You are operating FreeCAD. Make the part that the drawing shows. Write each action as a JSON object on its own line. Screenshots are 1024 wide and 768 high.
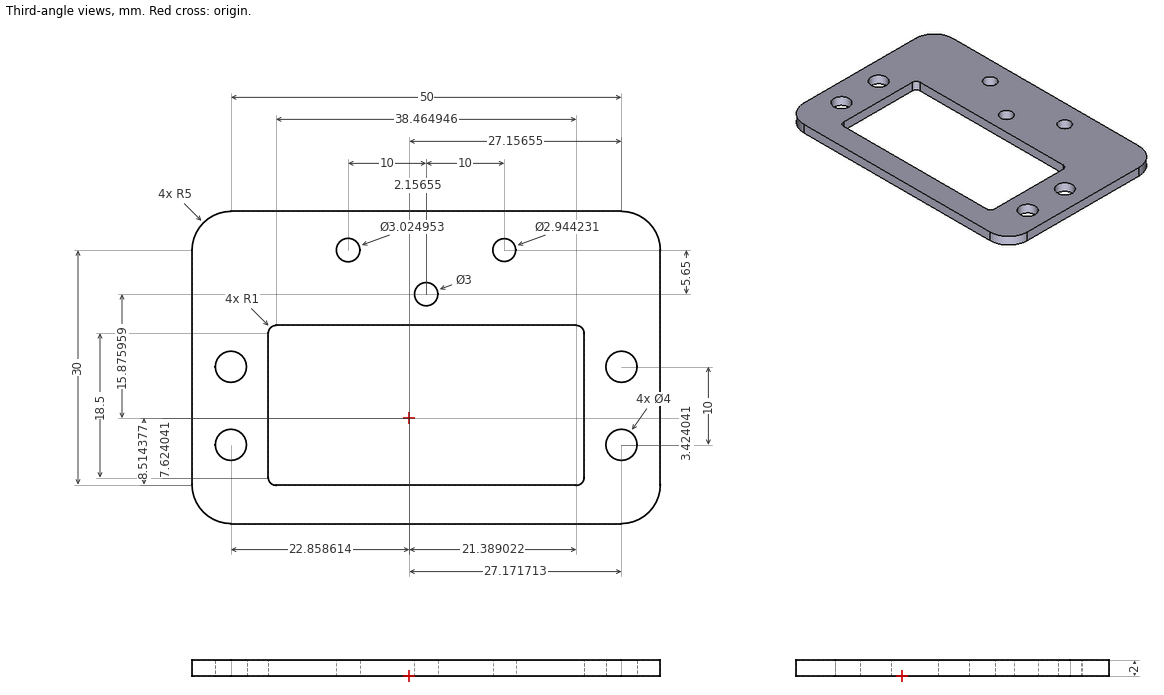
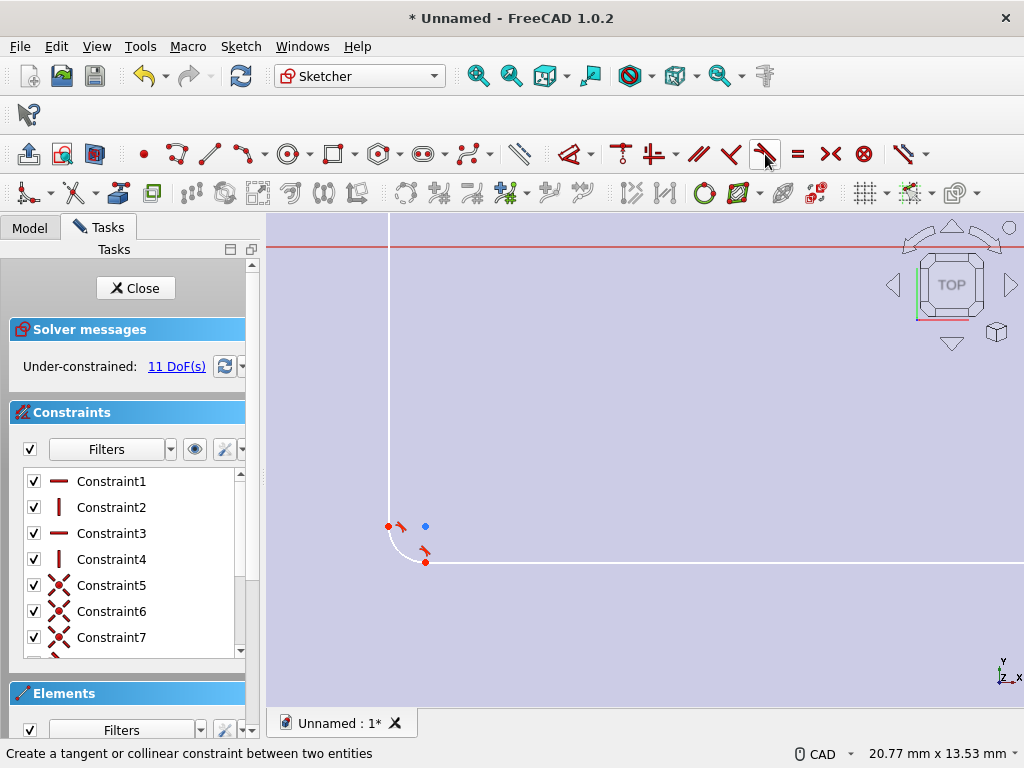
{"action": "scroll", "coordinate": [397, 549], "scroll_direction": "down", "scroll_amount": 7}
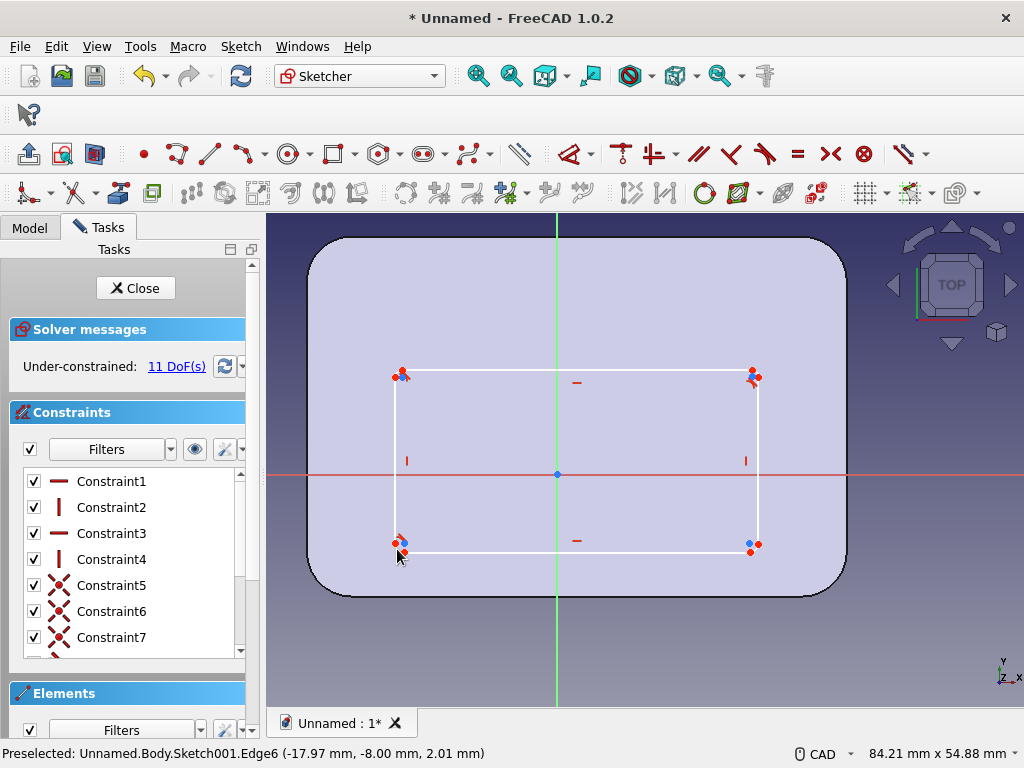
{"action": "left_click", "coordinate": [508, 553]}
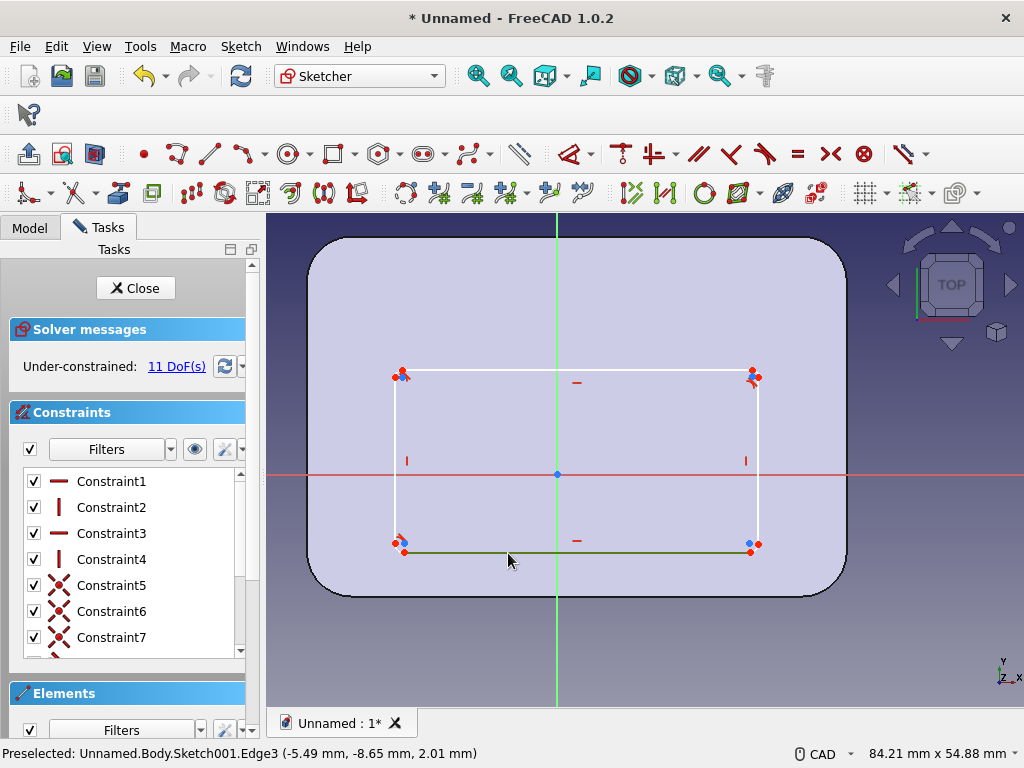
{"action": "scroll", "coordinate": [756, 550], "scroll_direction": "up", "scroll_amount": 4}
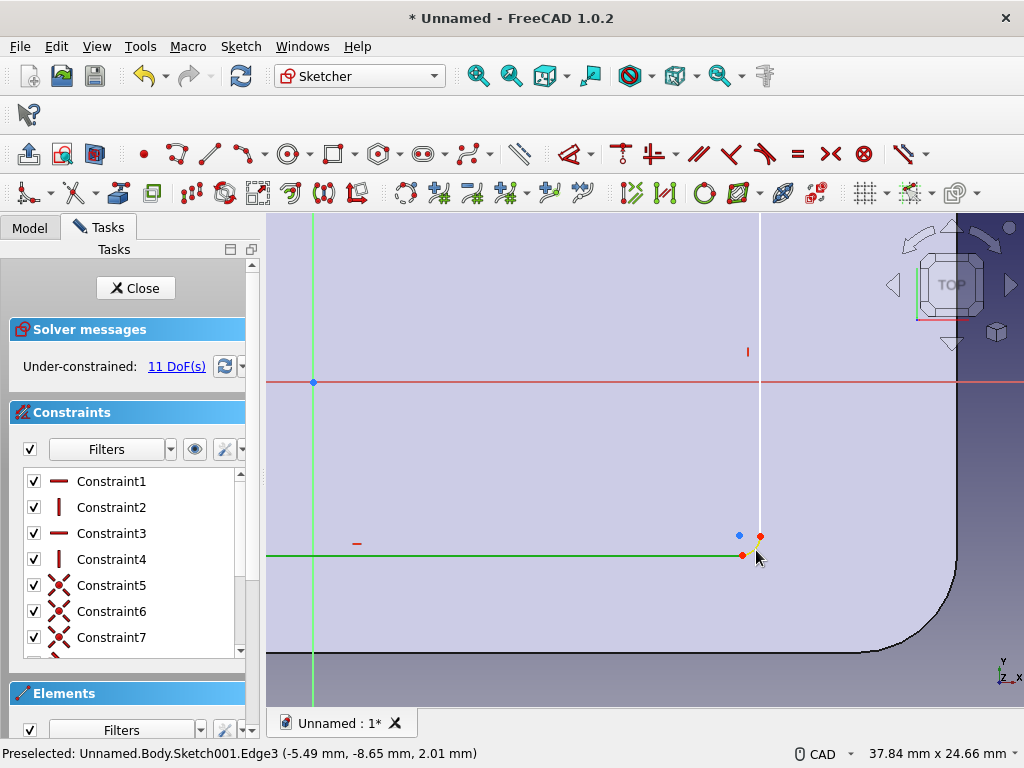
{"action": "left_click", "coordinate": [755, 549]}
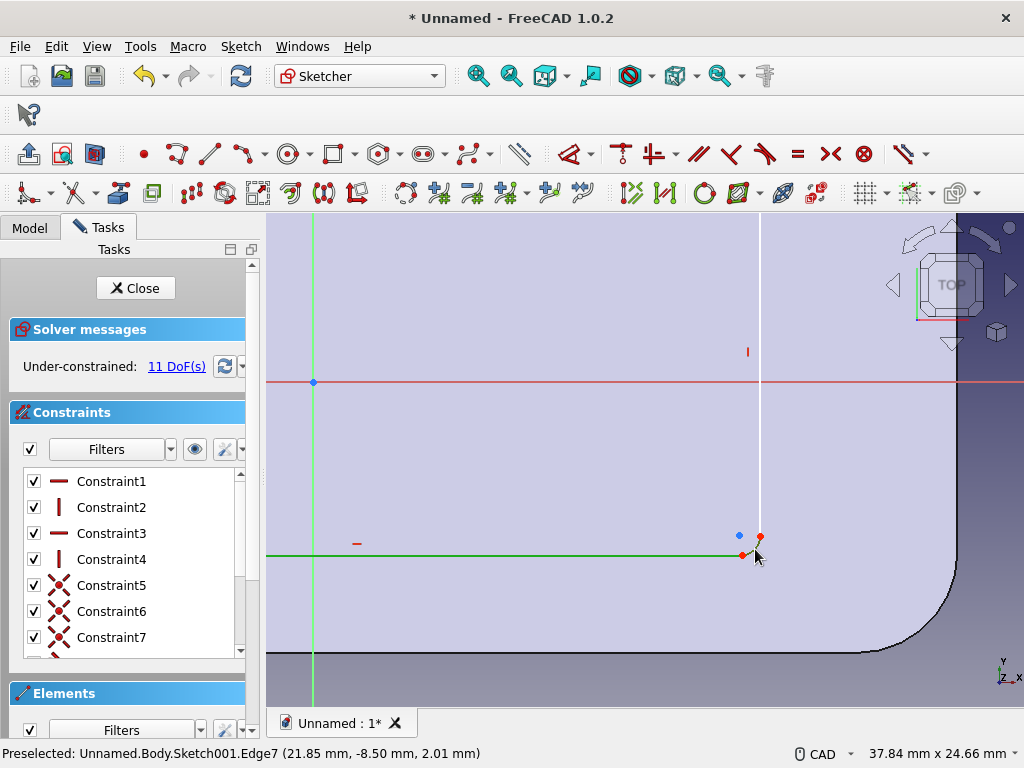
{"action": "left_click", "coordinate": [765, 154]}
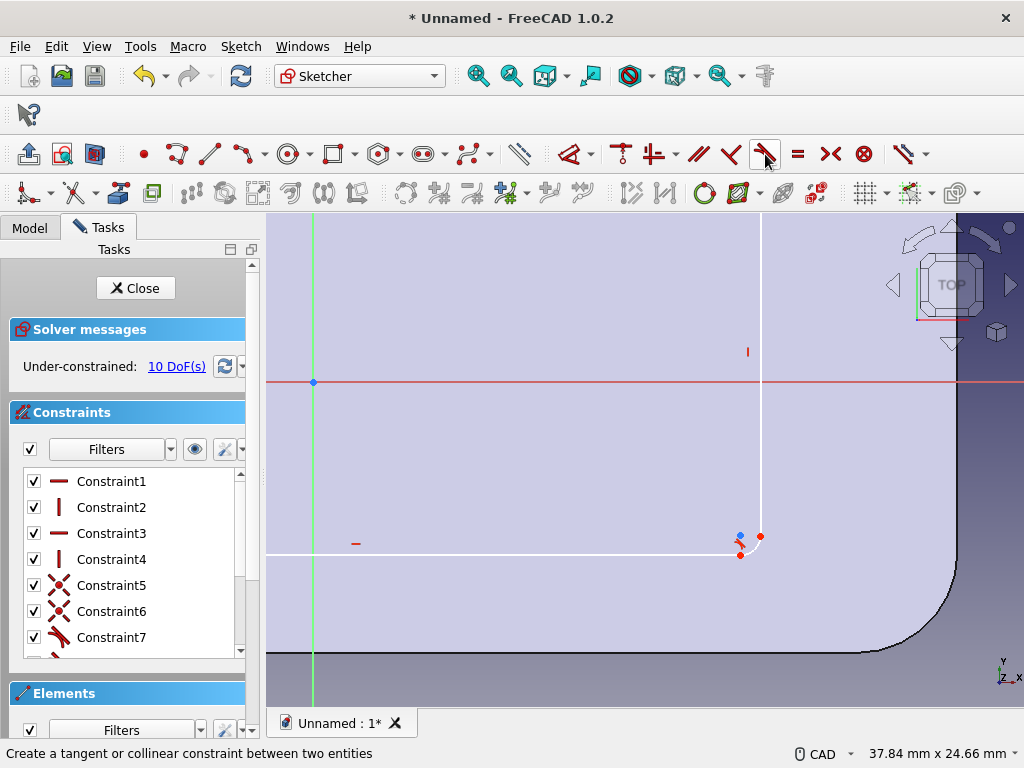
{"action": "left_click", "coordinate": [761, 425]}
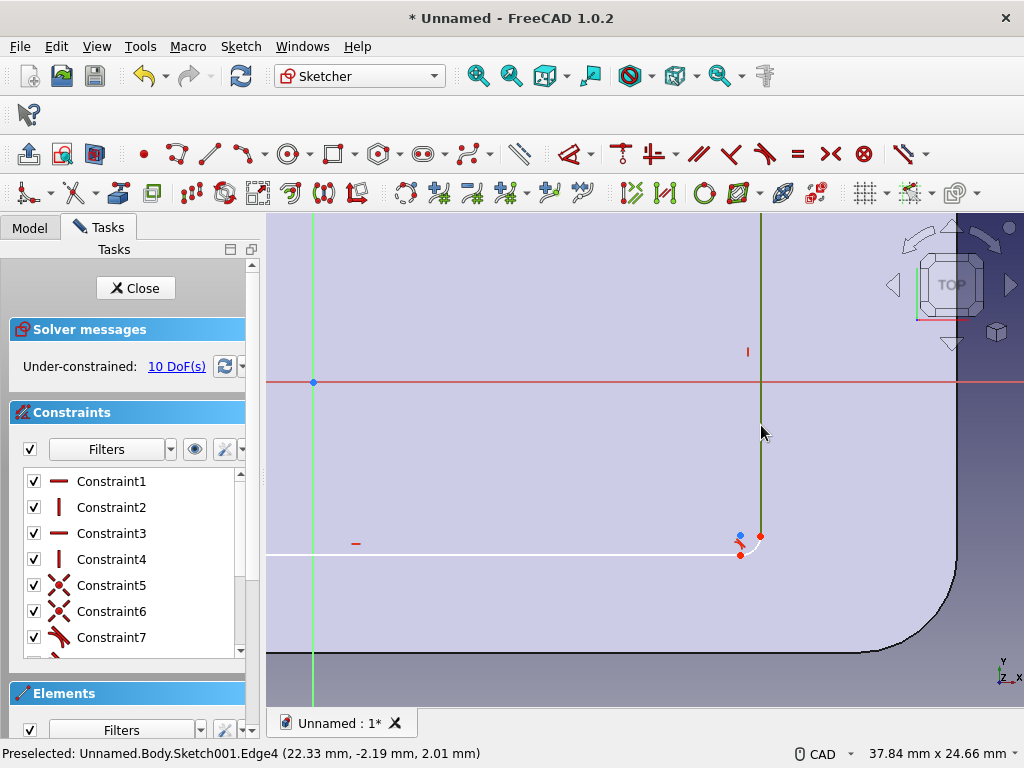
{"action": "scroll", "coordinate": [749, 553], "scroll_direction": "up", "scroll_amount": 2}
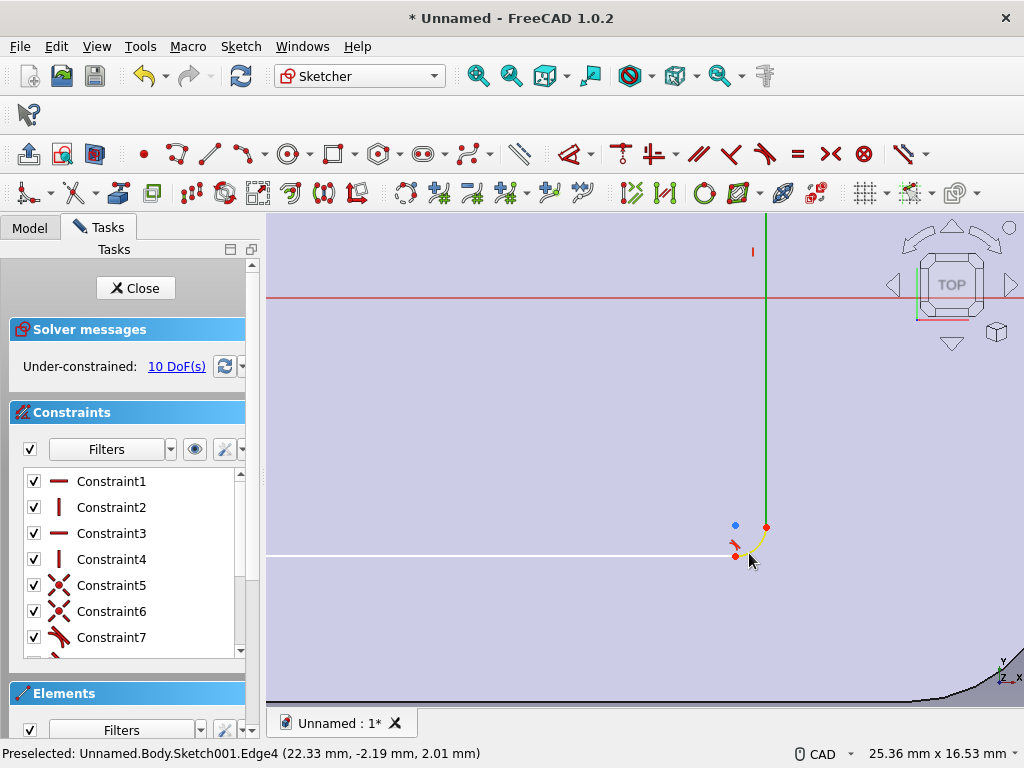
{"action": "left_click", "coordinate": [749, 553]}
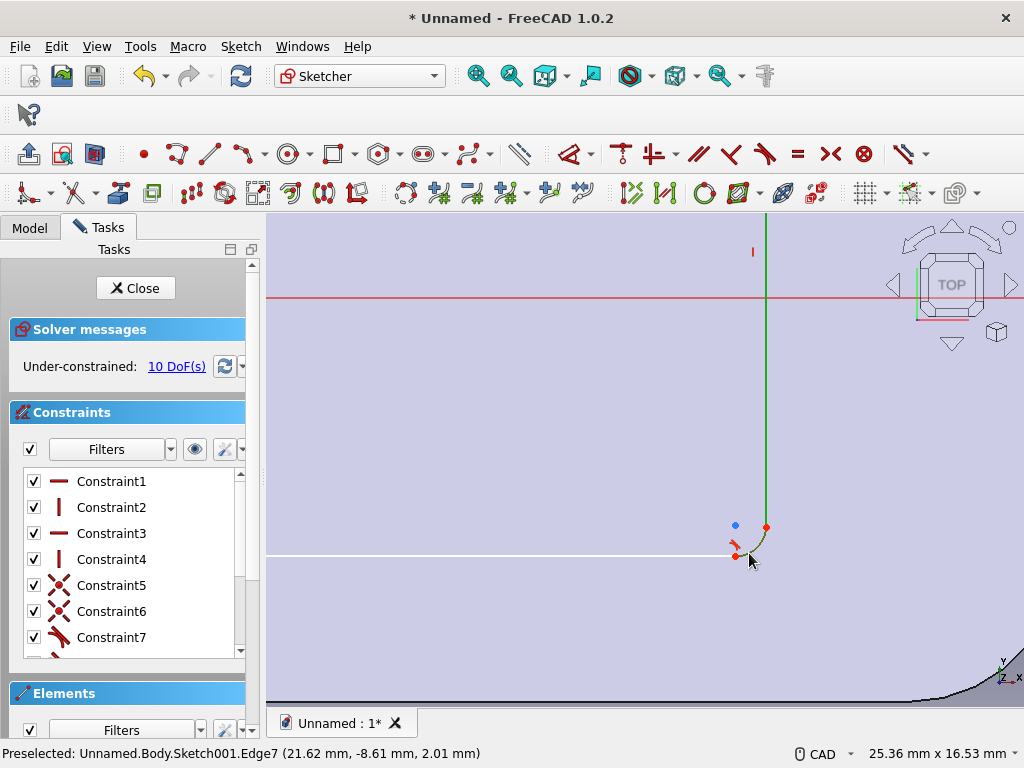
{"action": "left_click", "coordinate": [765, 154]}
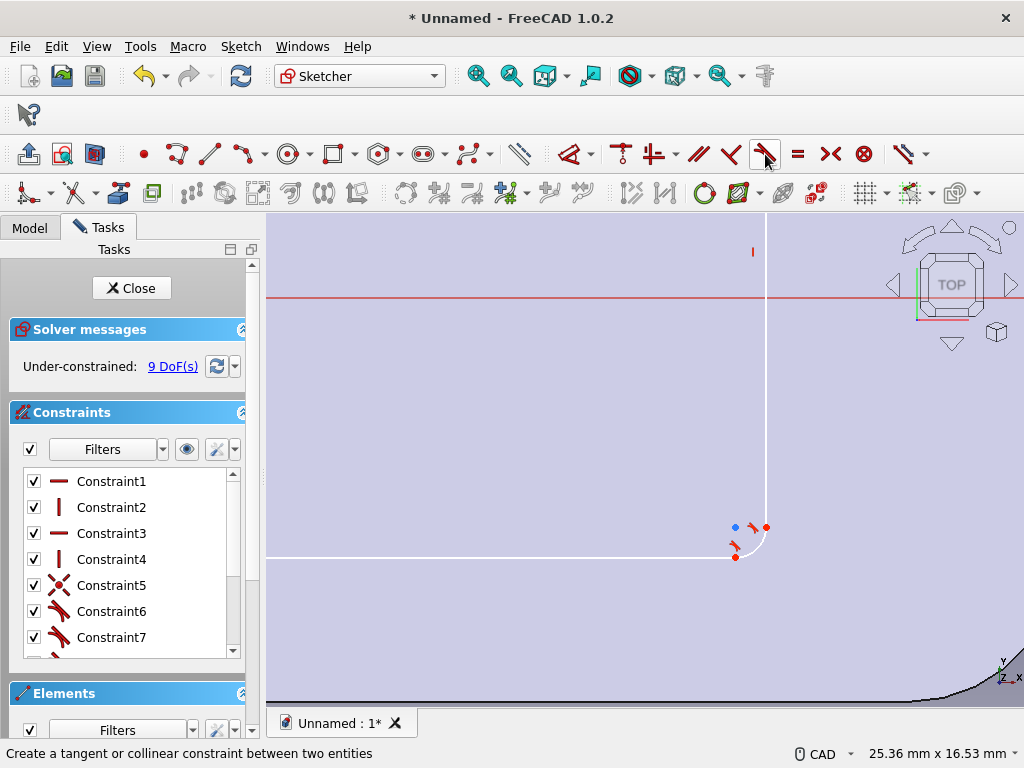
{"action": "left_click", "coordinate": [766, 362]}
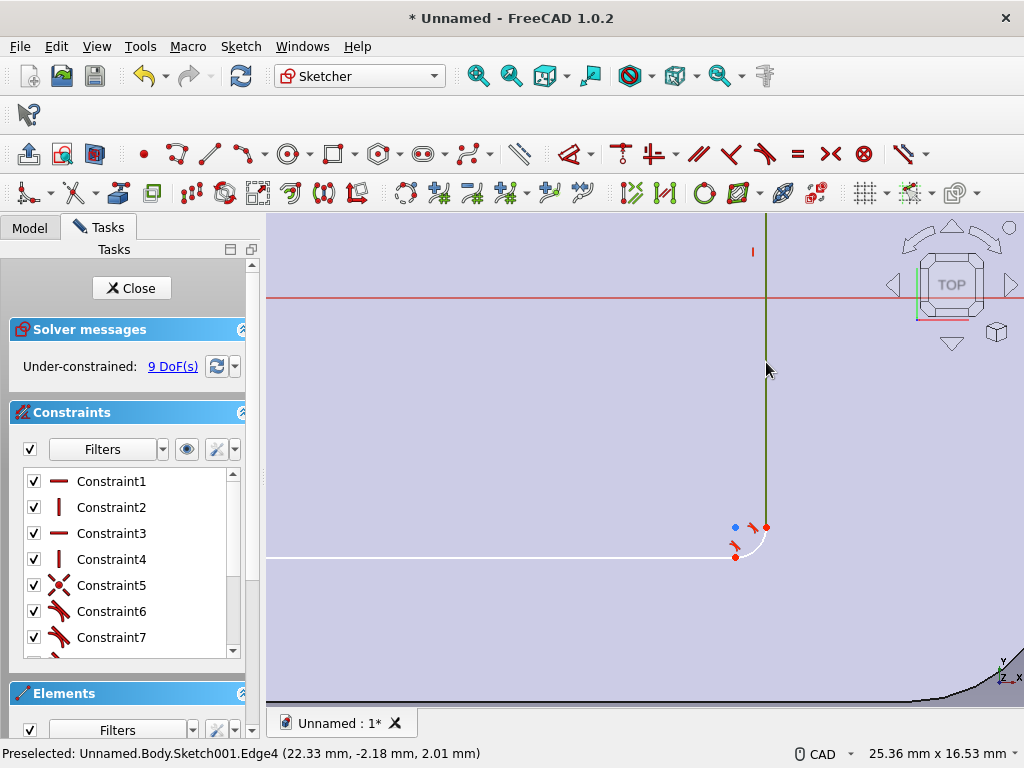
{"action": "scroll", "coordinate": [755, 551], "scroll_direction": "down", "scroll_amount": 6}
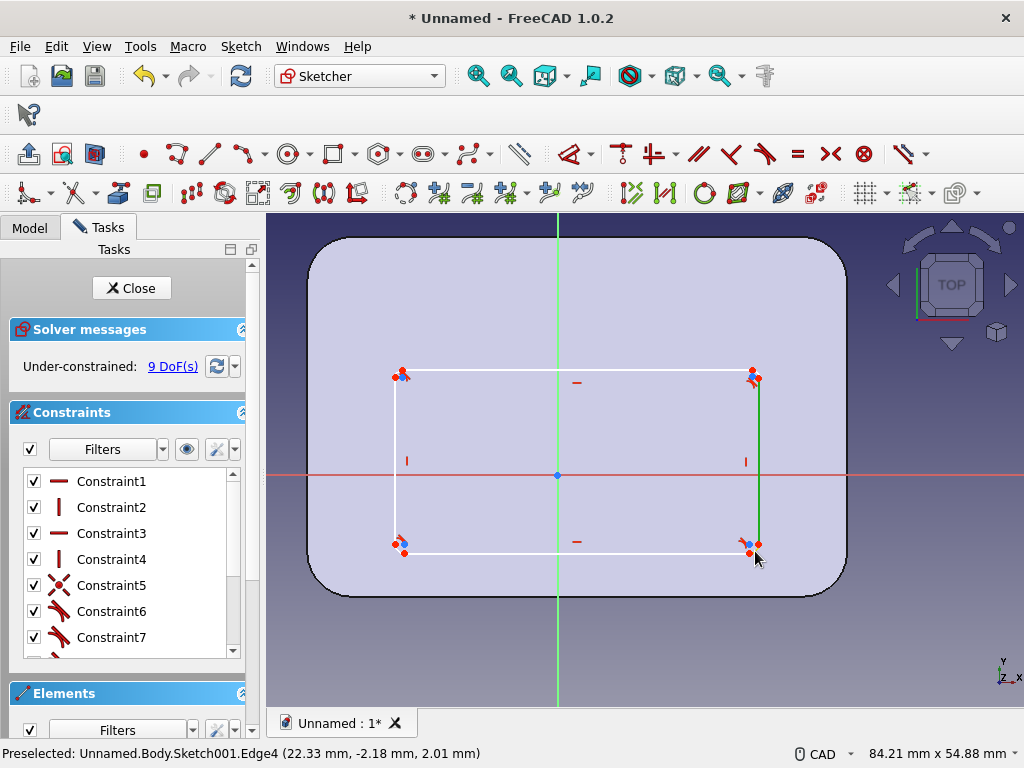
{"action": "scroll", "coordinate": [759, 375], "scroll_direction": "up", "scroll_amount": 7}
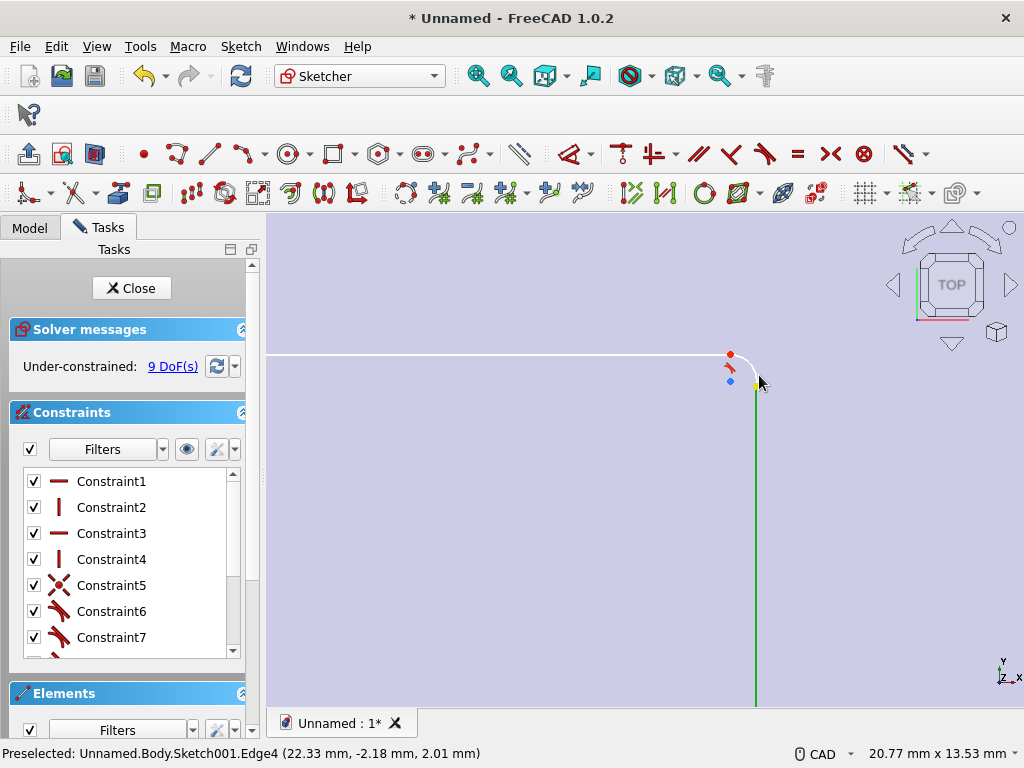
{"action": "left_click", "coordinate": [755, 373]}